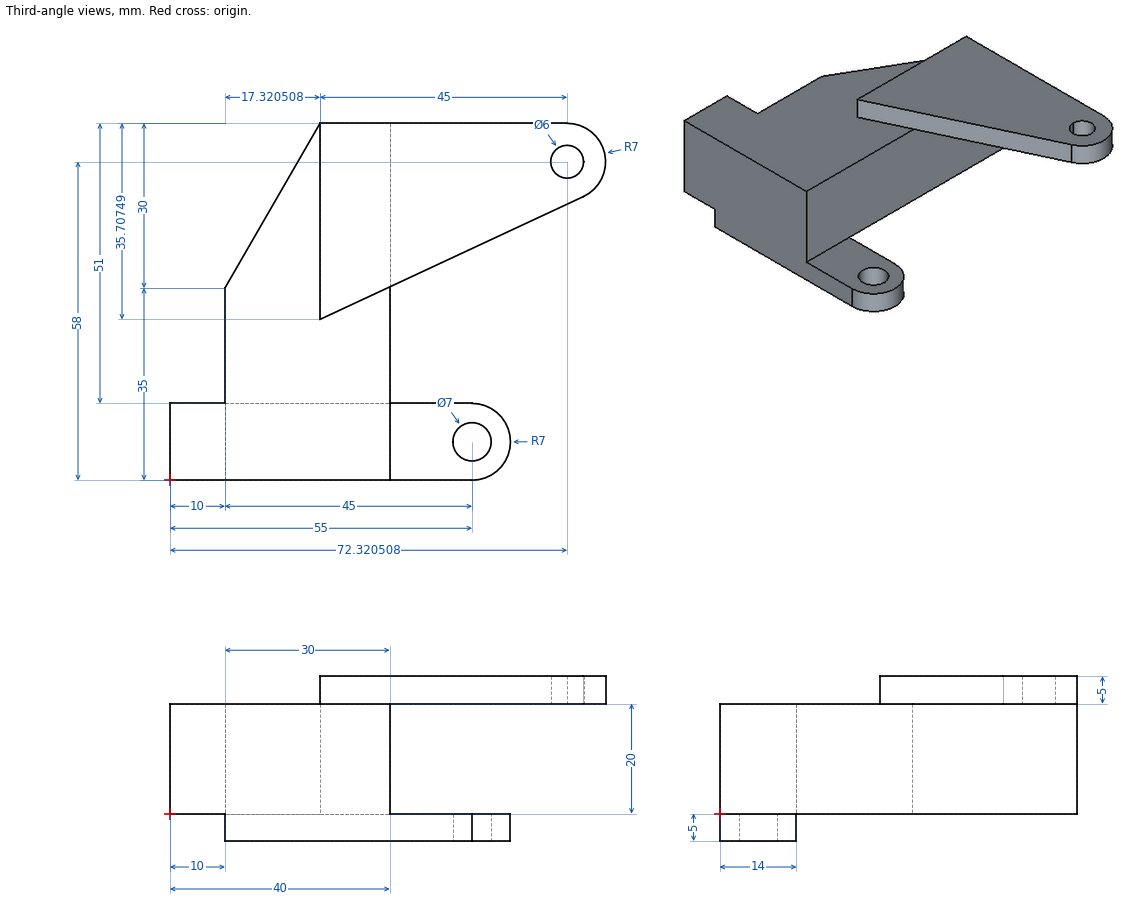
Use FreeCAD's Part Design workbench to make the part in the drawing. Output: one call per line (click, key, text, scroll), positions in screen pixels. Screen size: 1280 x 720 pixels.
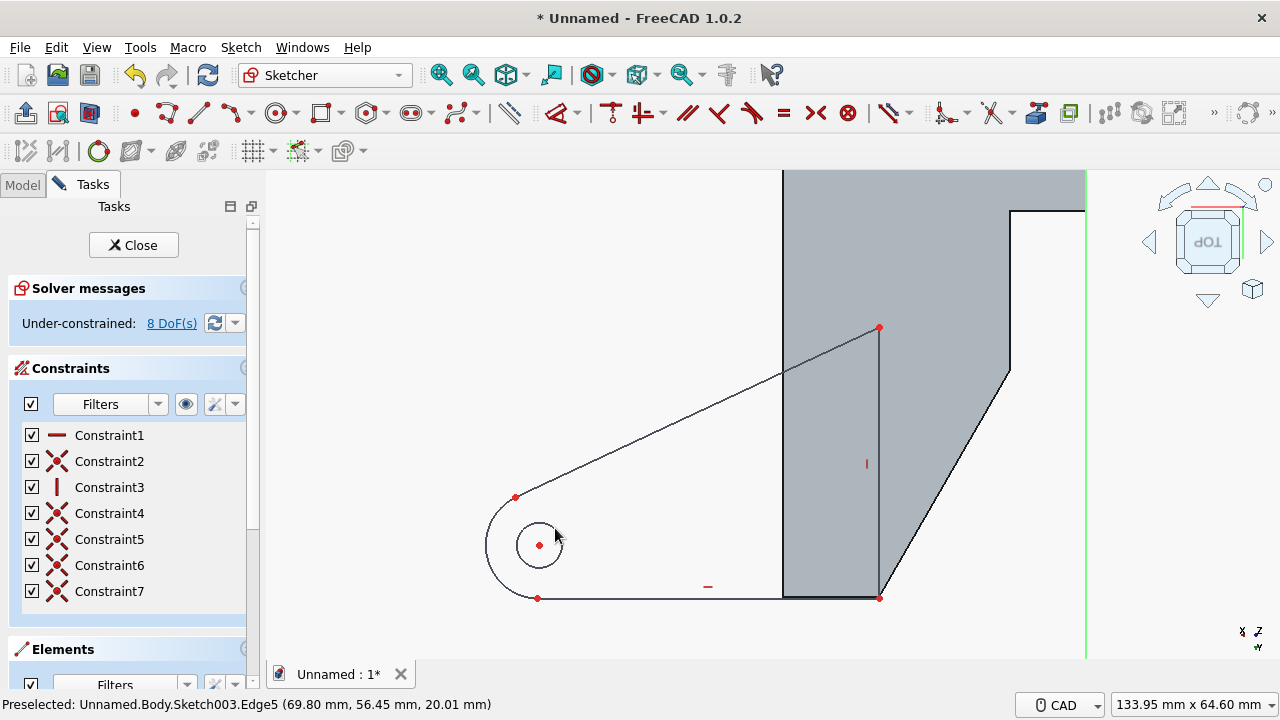
click(640, 599)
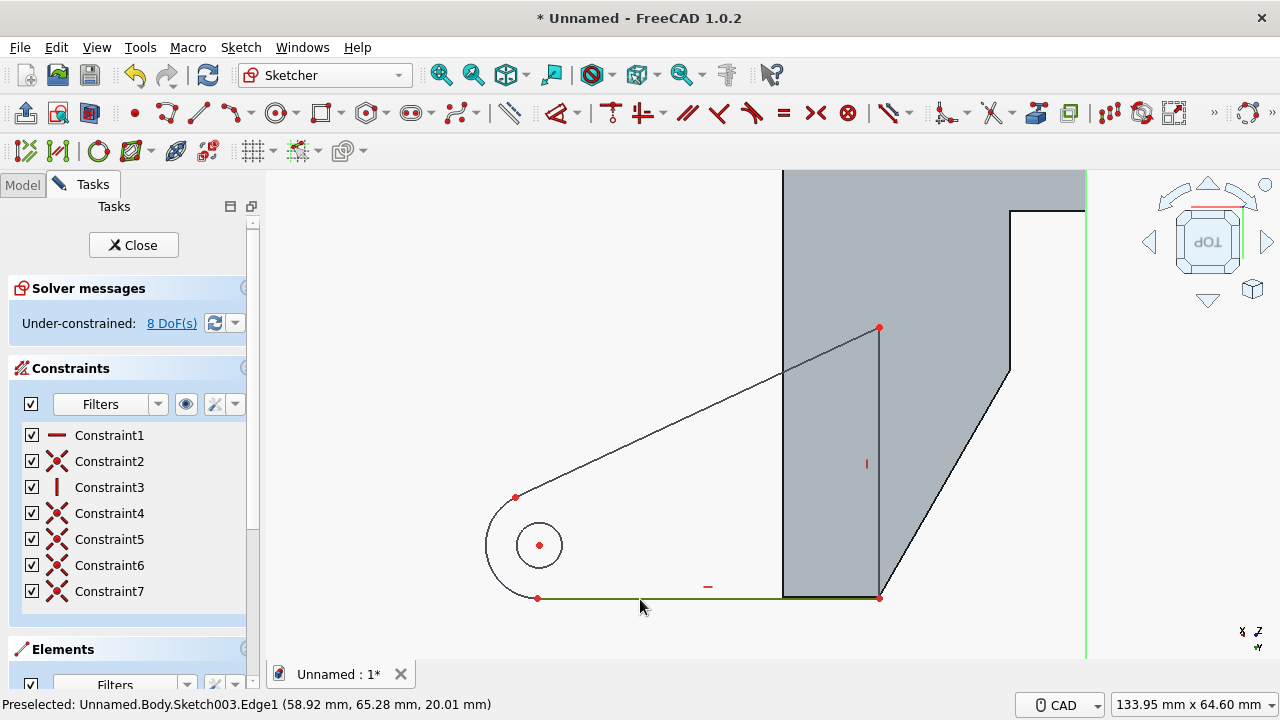
click(488, 529)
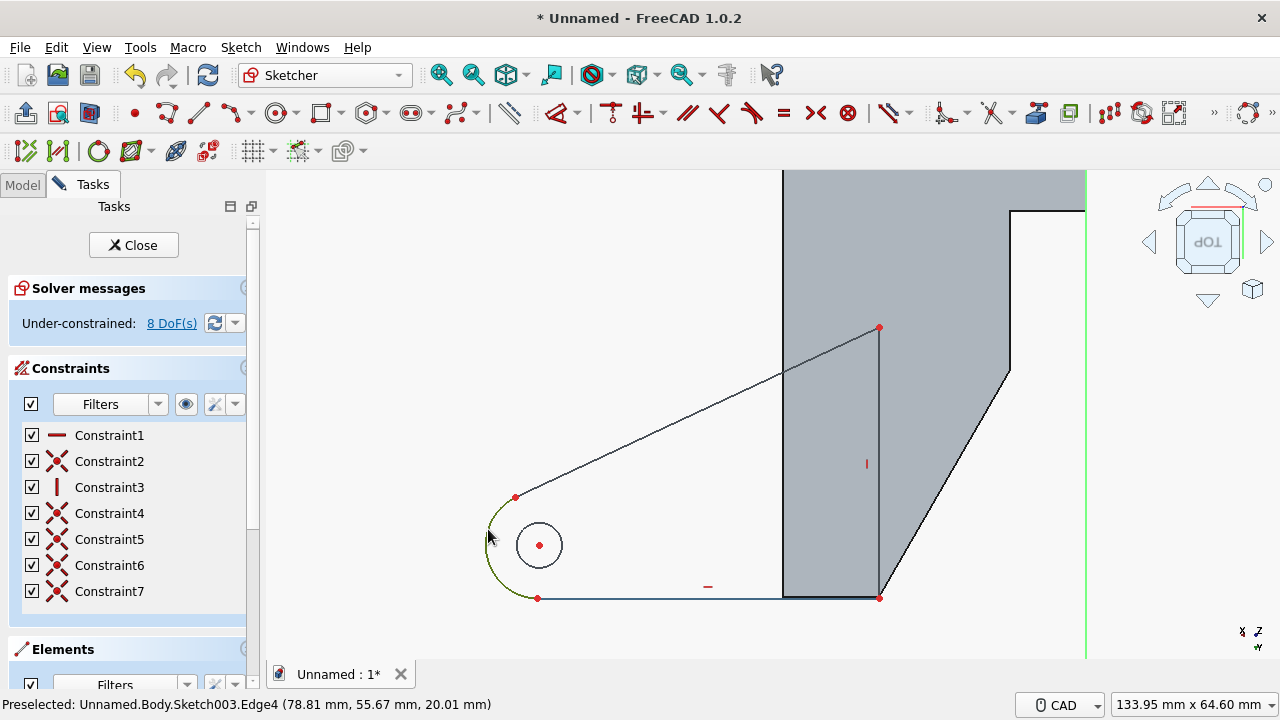
click(752, 114)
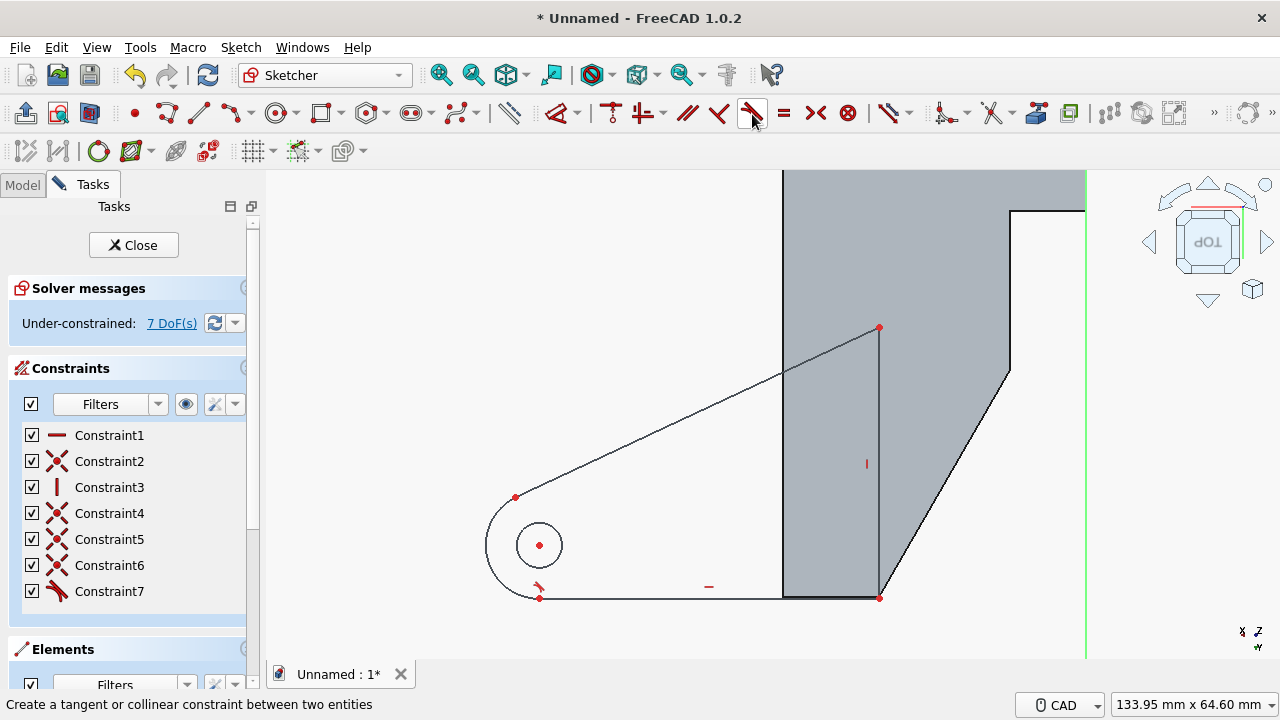
click(770, 378)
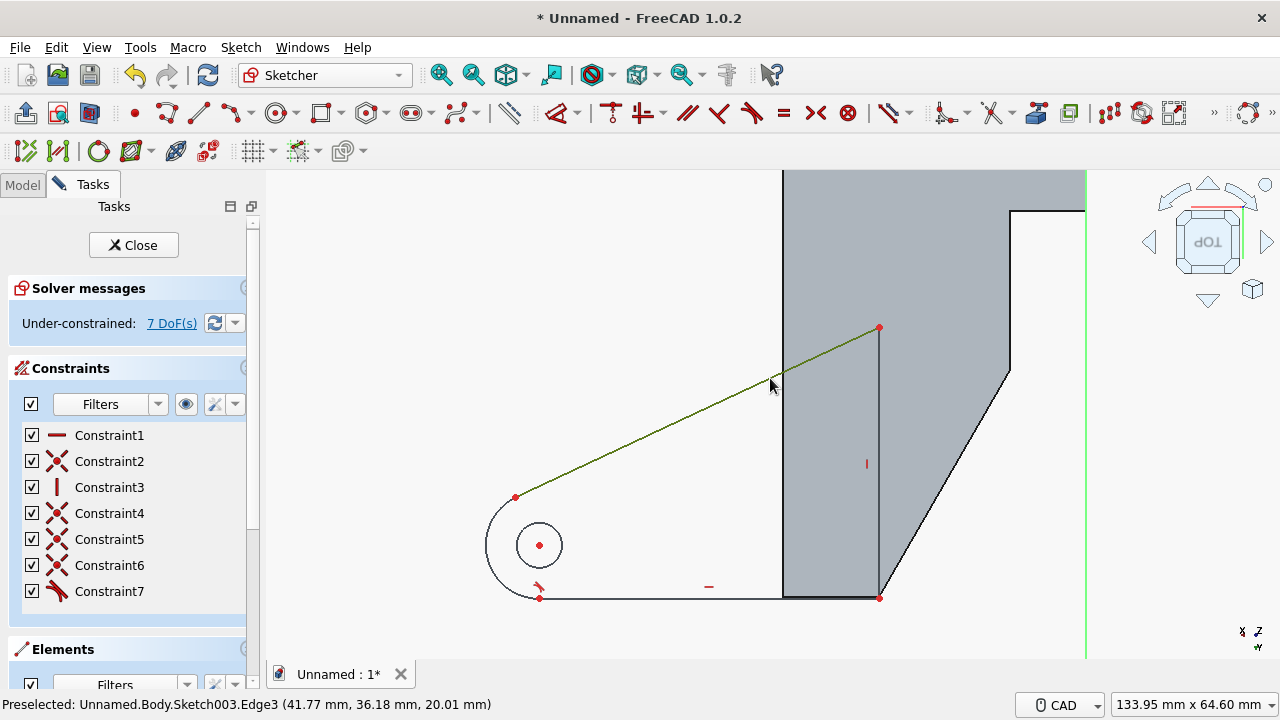
click(488, 529)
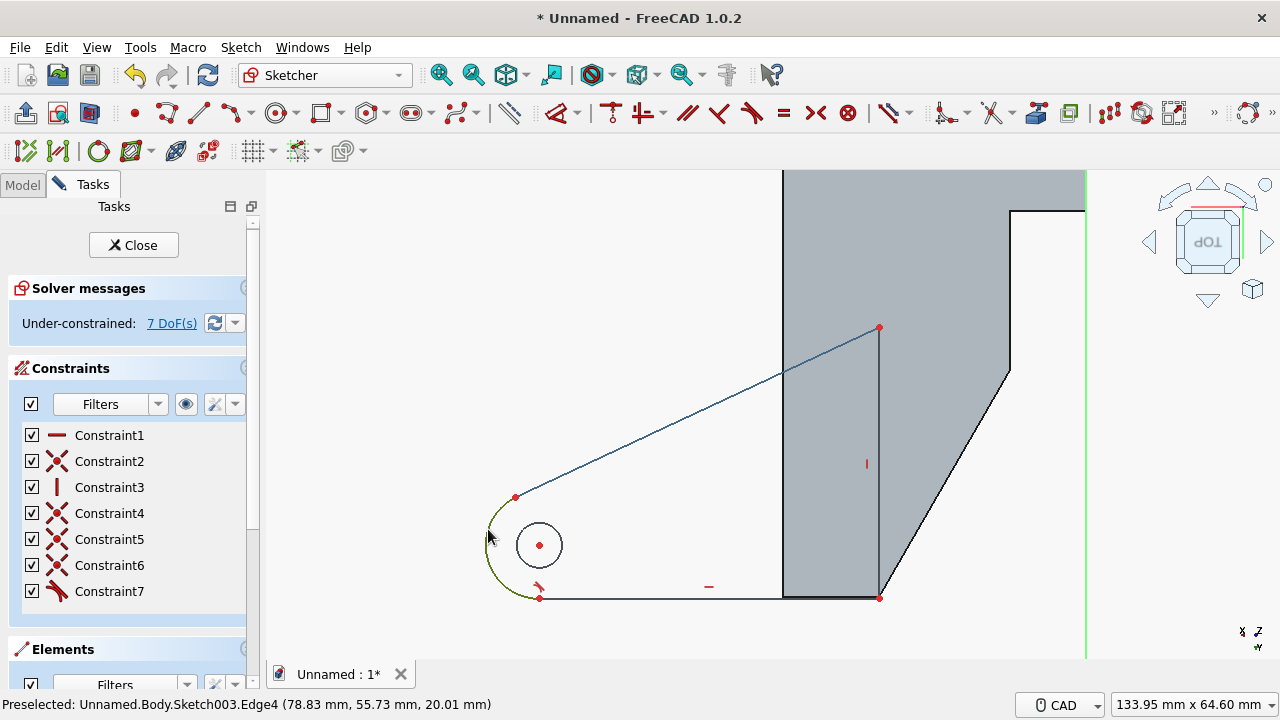
key(t)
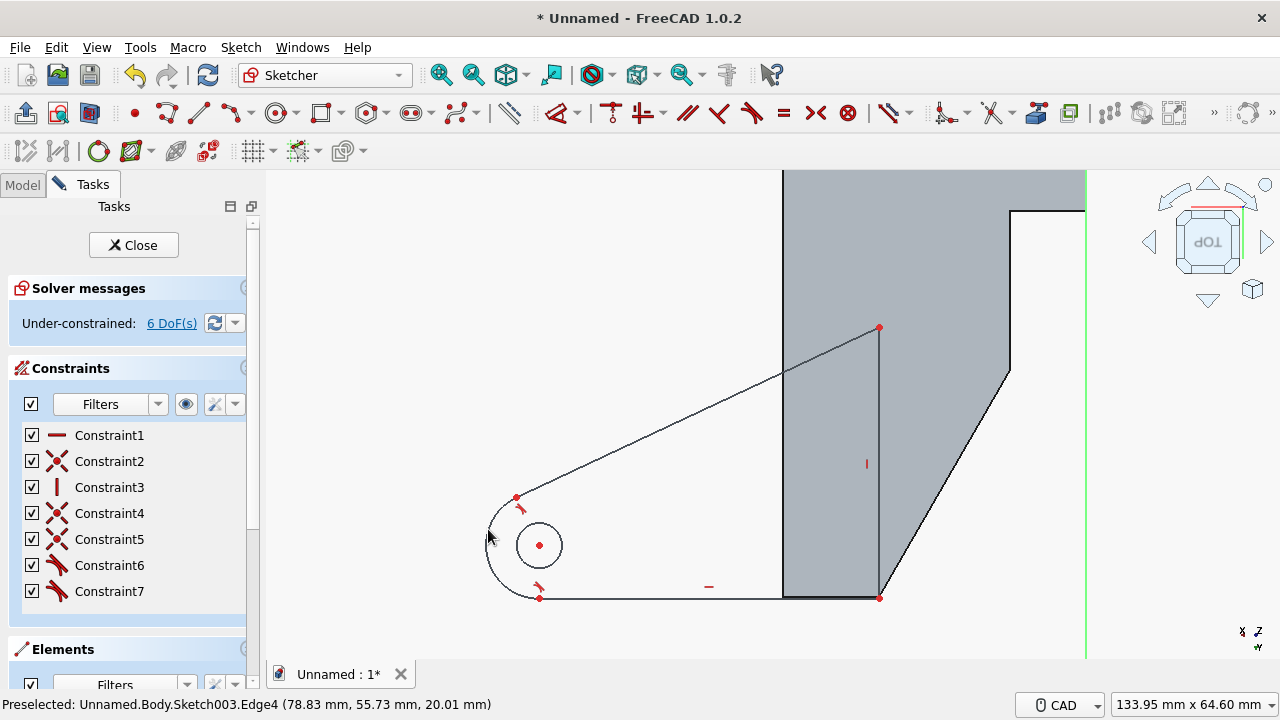
click(556, 114)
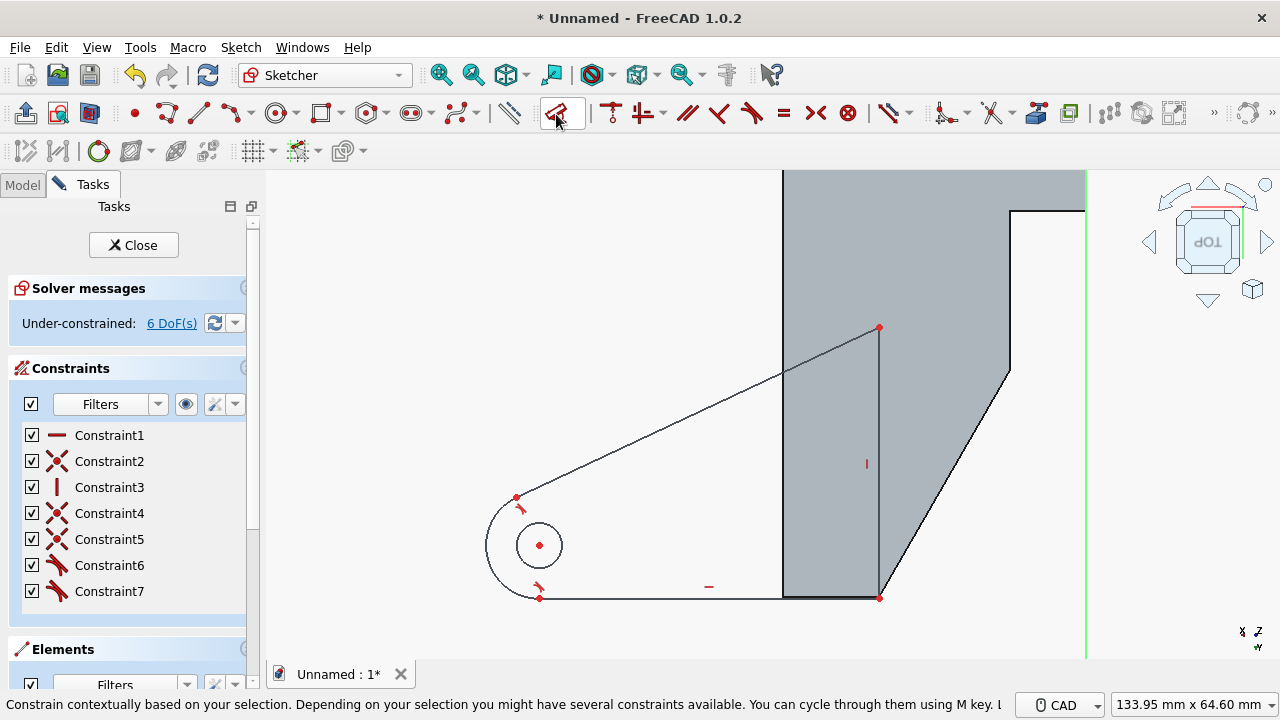
click(489, 529)
click(459, 519)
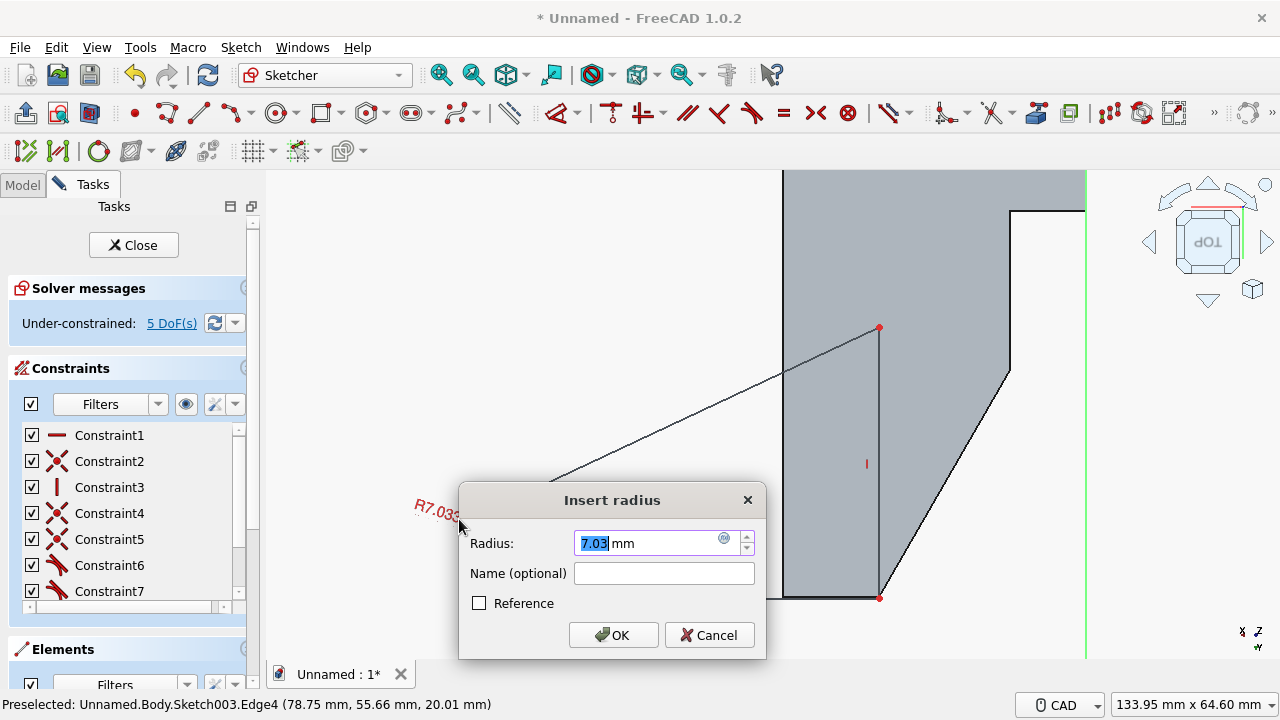
text(7)
key(Return)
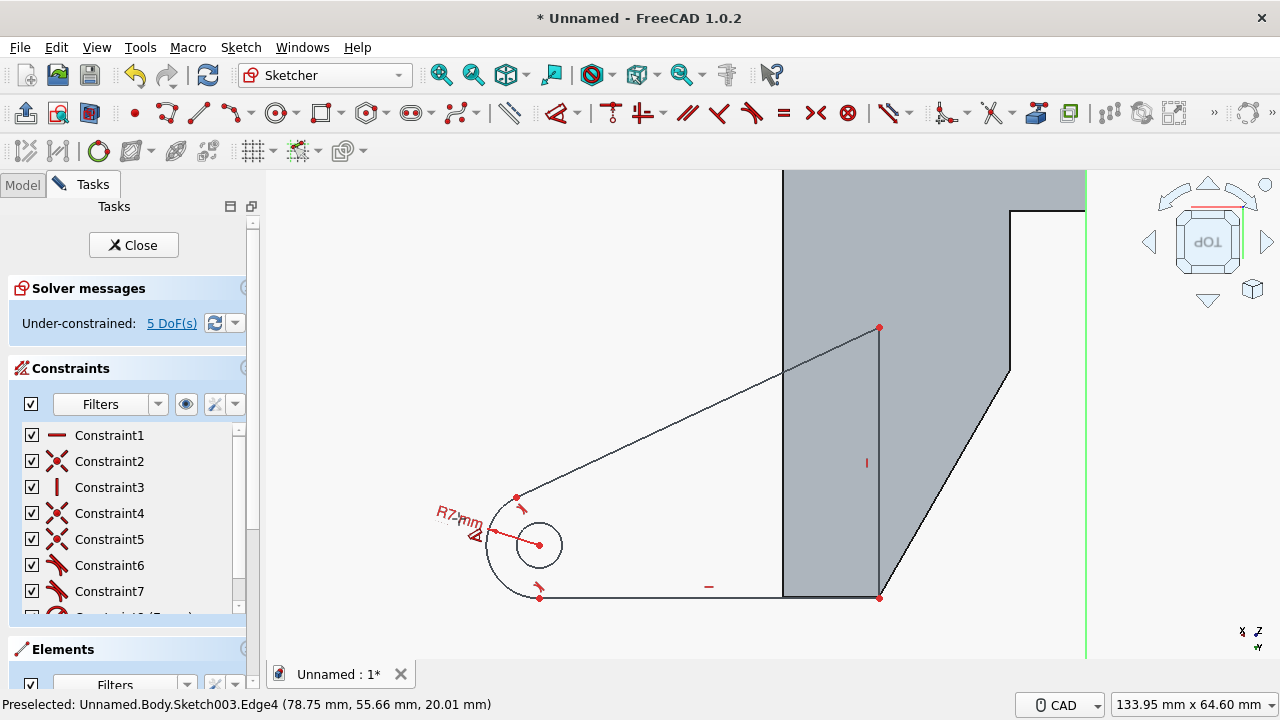
click(555, 529)
click(577, 506)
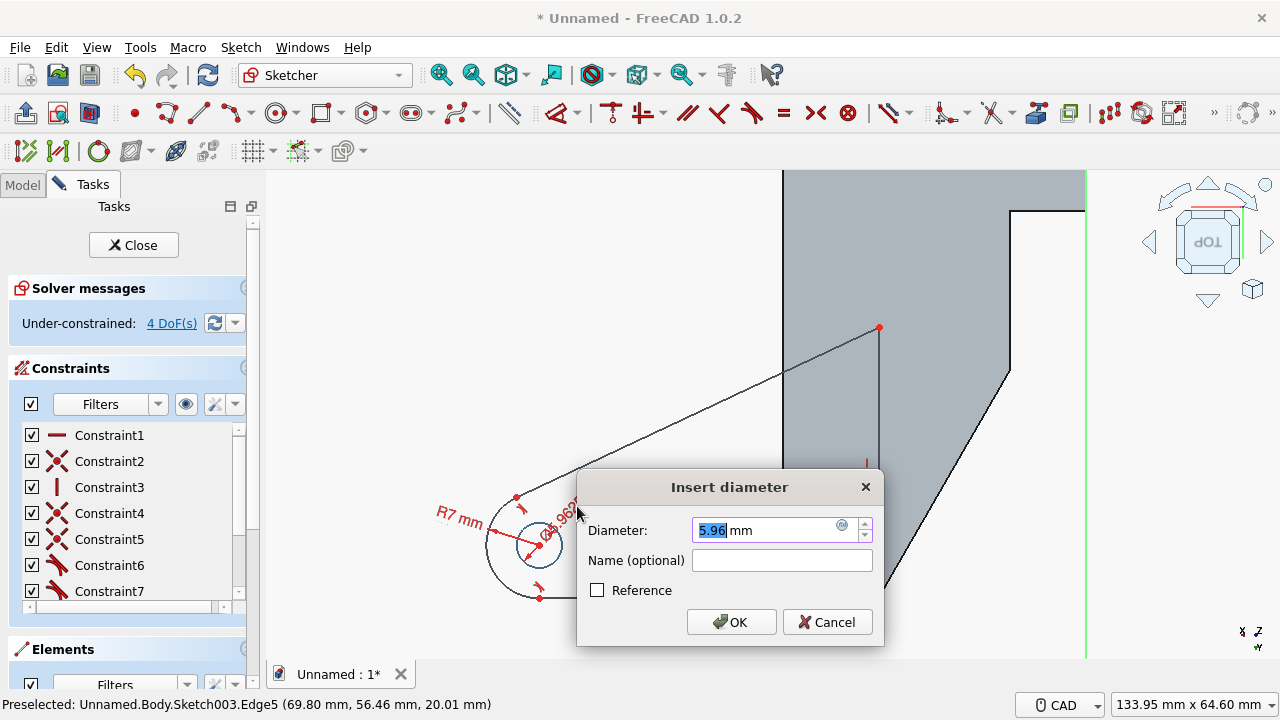
text(6)
key(Return)